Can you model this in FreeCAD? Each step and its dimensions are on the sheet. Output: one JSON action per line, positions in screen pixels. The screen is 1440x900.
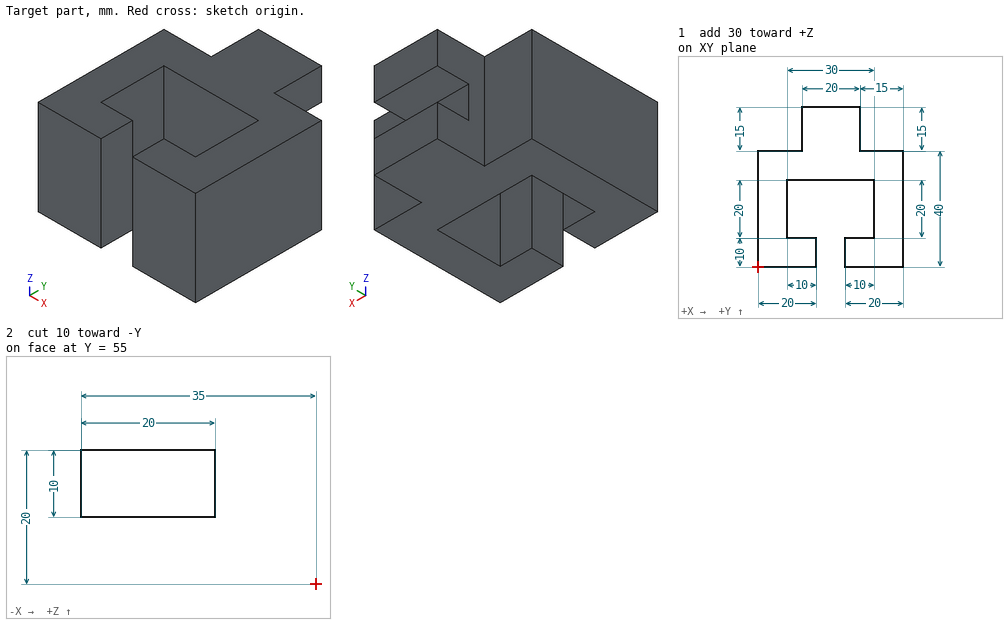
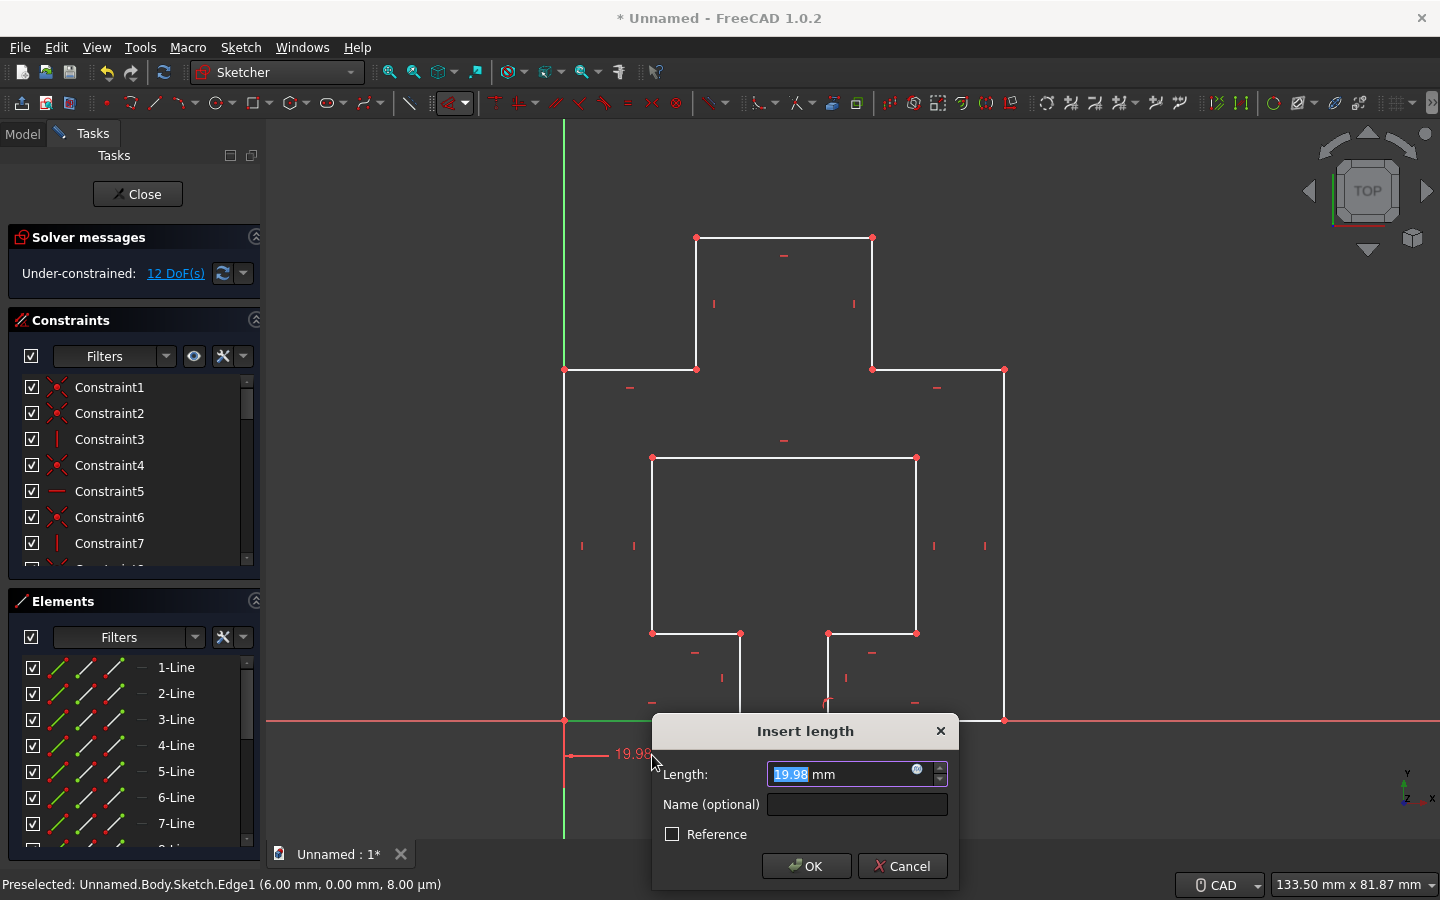
{"action": "type", "text": "20"}
{"action": "key", "text": "Return"}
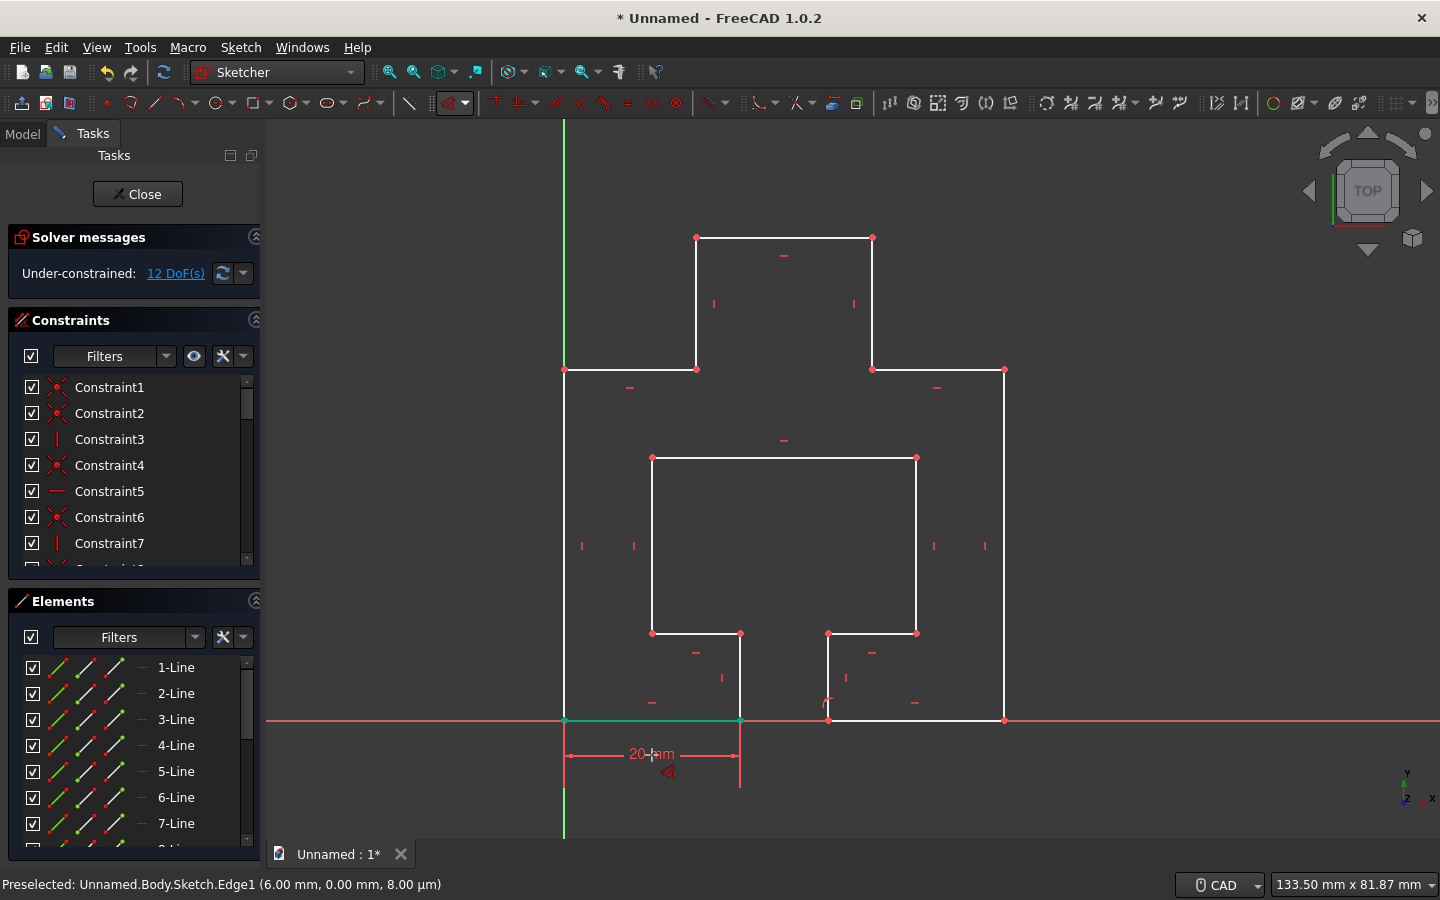
{"action": "left_click", "coordinate": [740, 695]}
{"action": "left_click", "coordinate": [706, 677]}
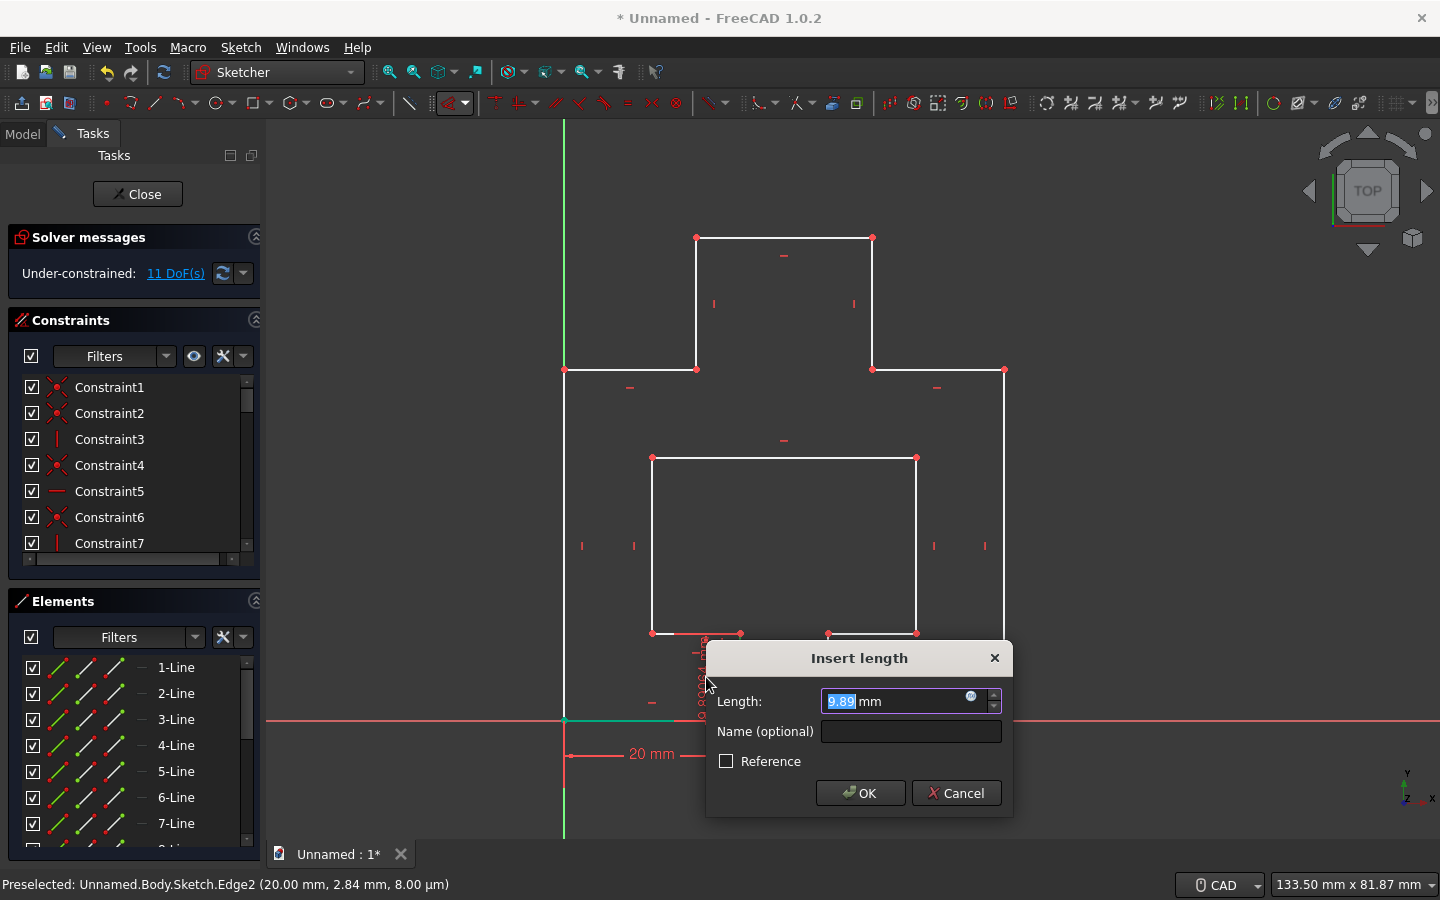
{"action": "type", "text": "10"}
{"action": "key", "text": "Return"}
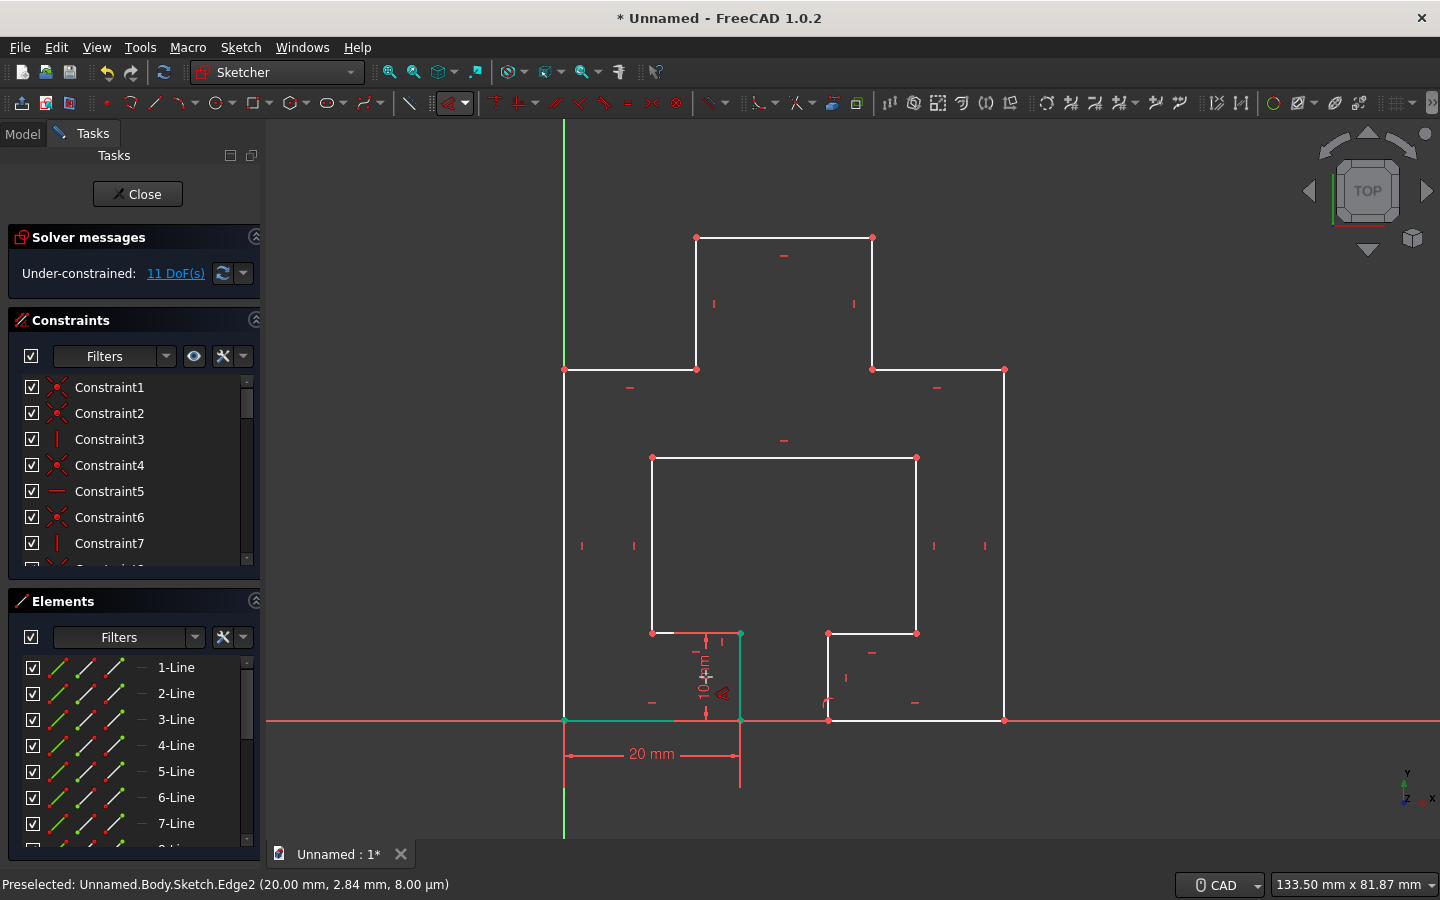
{"action": "left_click", "coordinate": [714, 633]}
{"action": "left_click", "coordinate": [696, 599]}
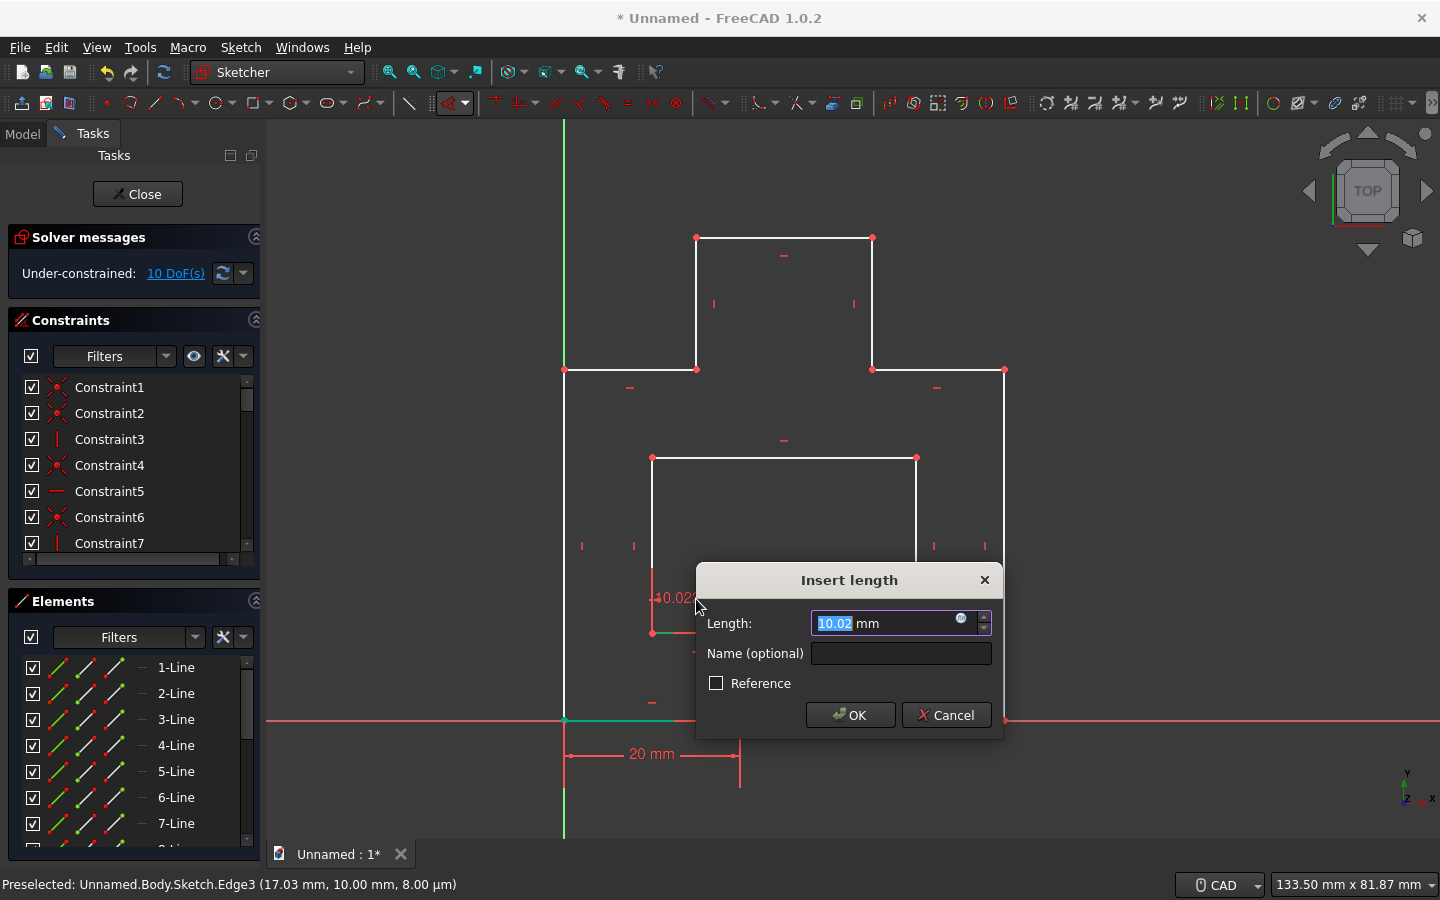
{"action": "type", "text": "10"}
{"action": "key", "text": "Return"}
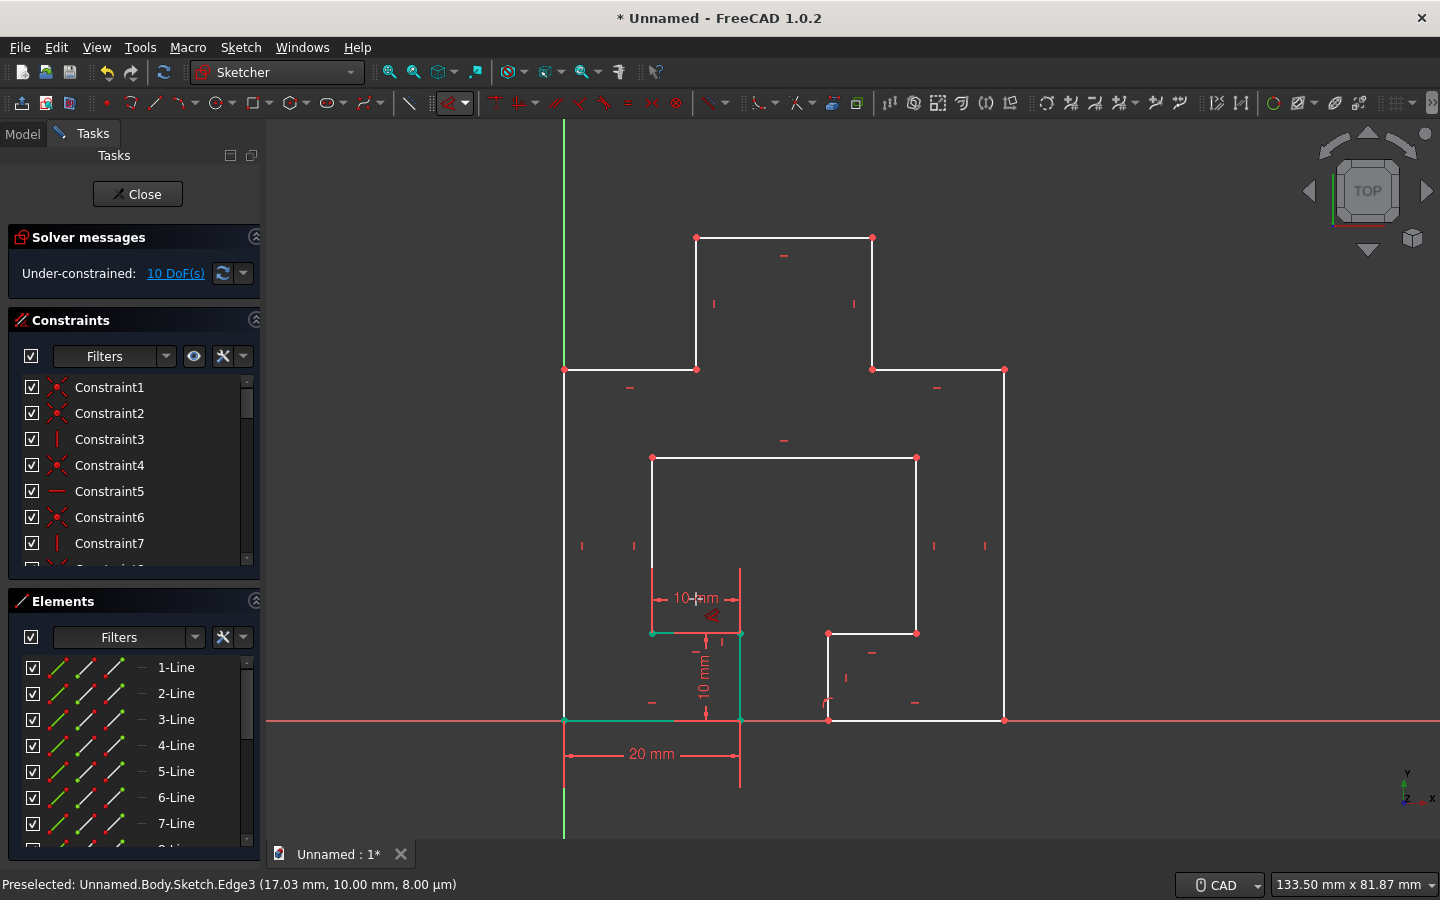
{"action": "left_click", "coordinate": [652, 581]}
{"action": "left_click", "coordinate": [618, 546]}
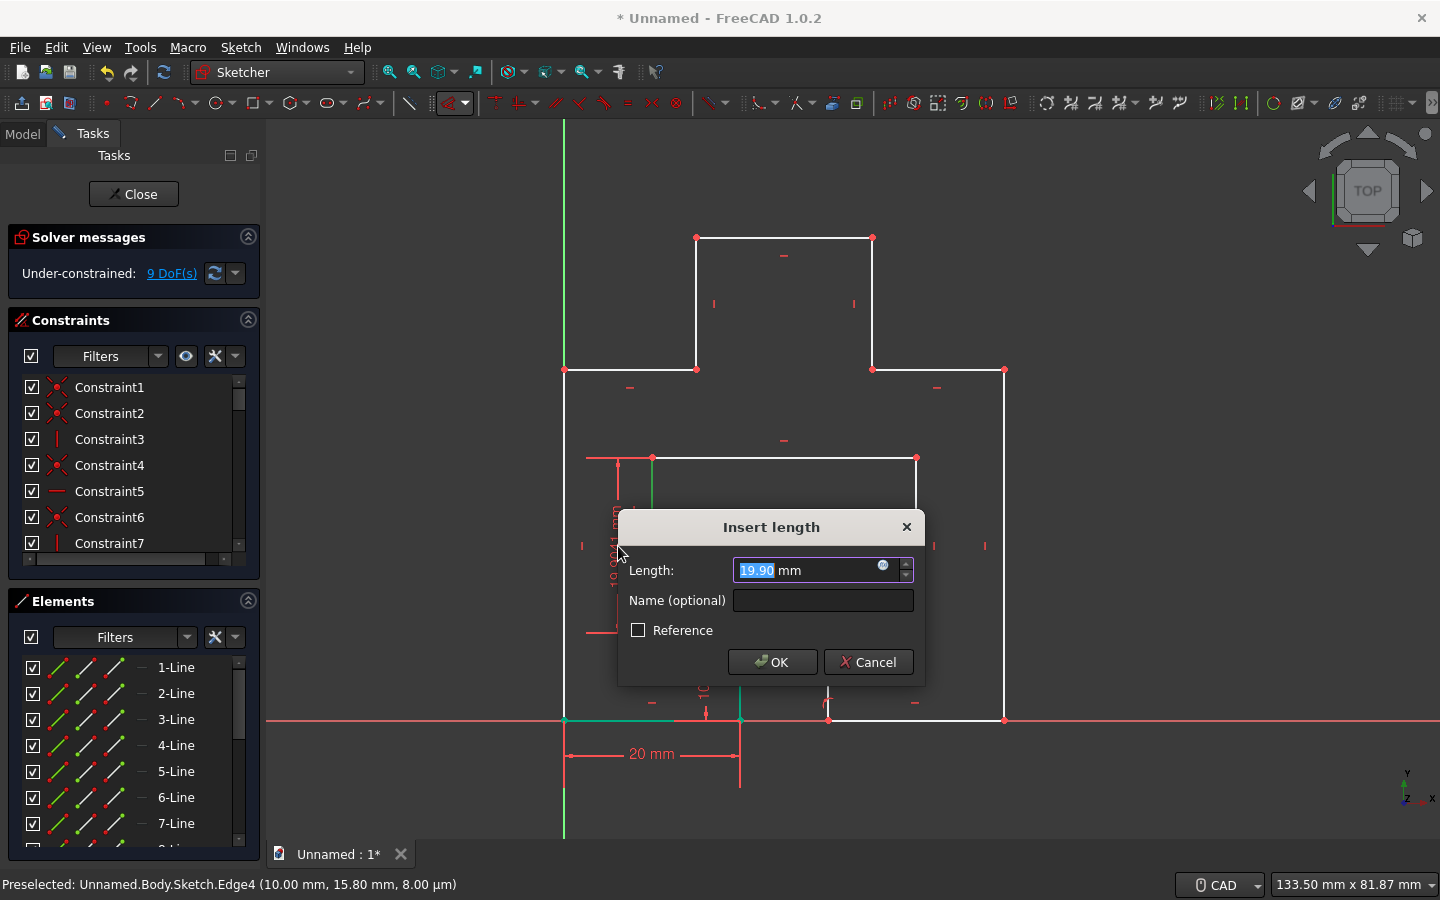
{"action": "type", "text": "20"}
{"action": "key", "text": "Return"}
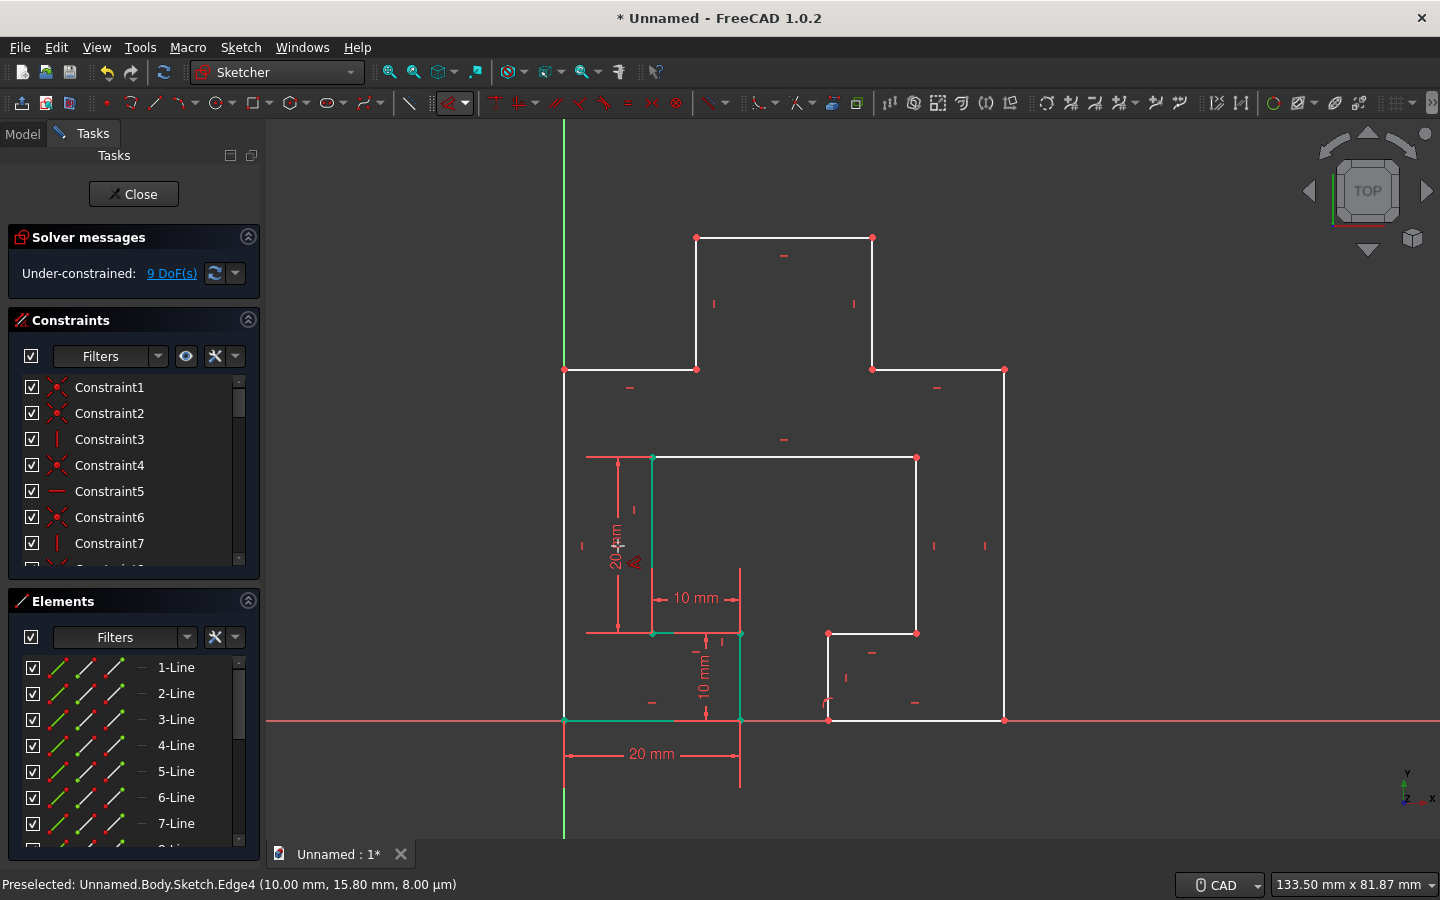
{"action": "left_click", "coordinate": [731, 457]}
{"action": "left_click", "coordinate": [784, 423]}